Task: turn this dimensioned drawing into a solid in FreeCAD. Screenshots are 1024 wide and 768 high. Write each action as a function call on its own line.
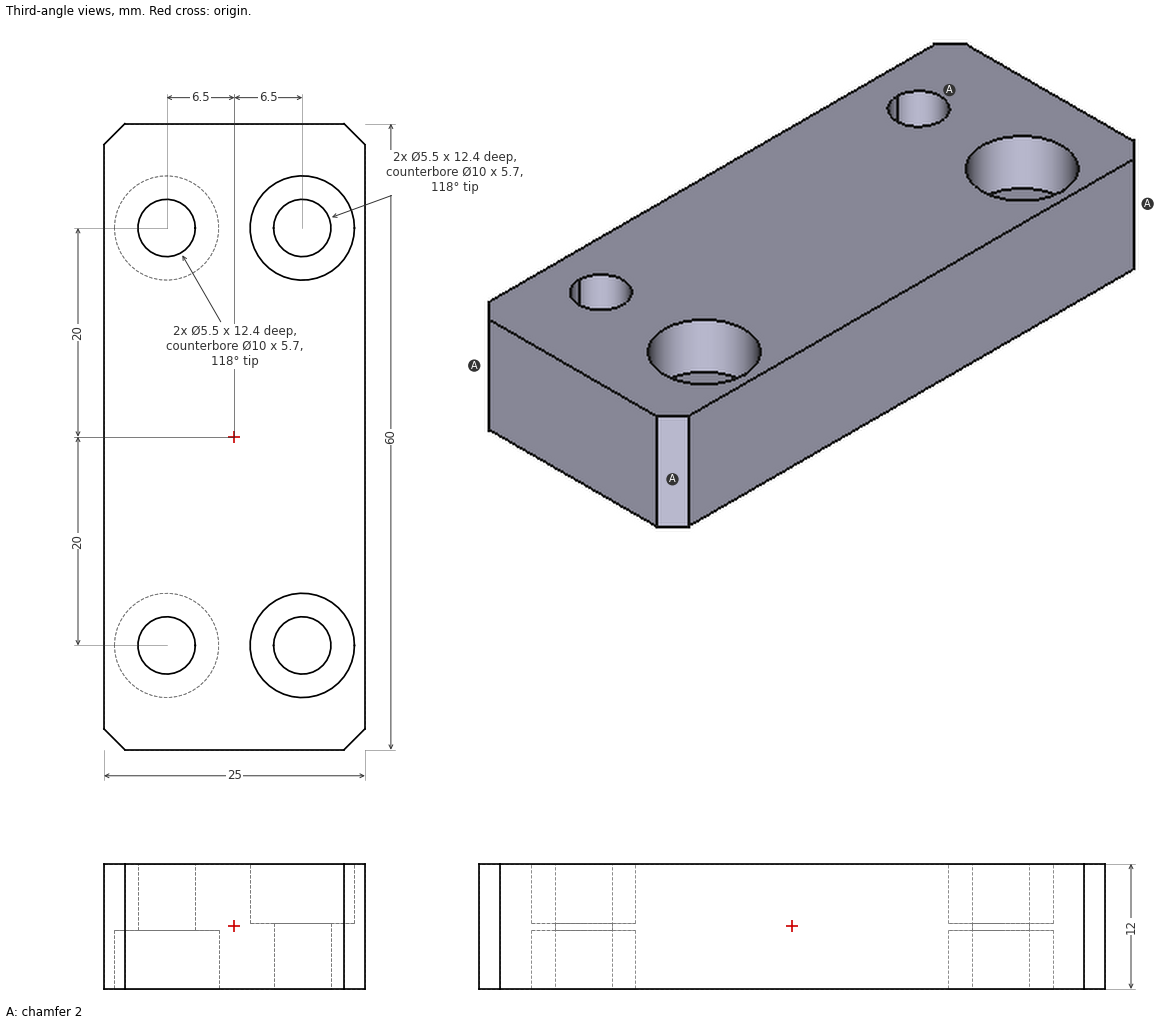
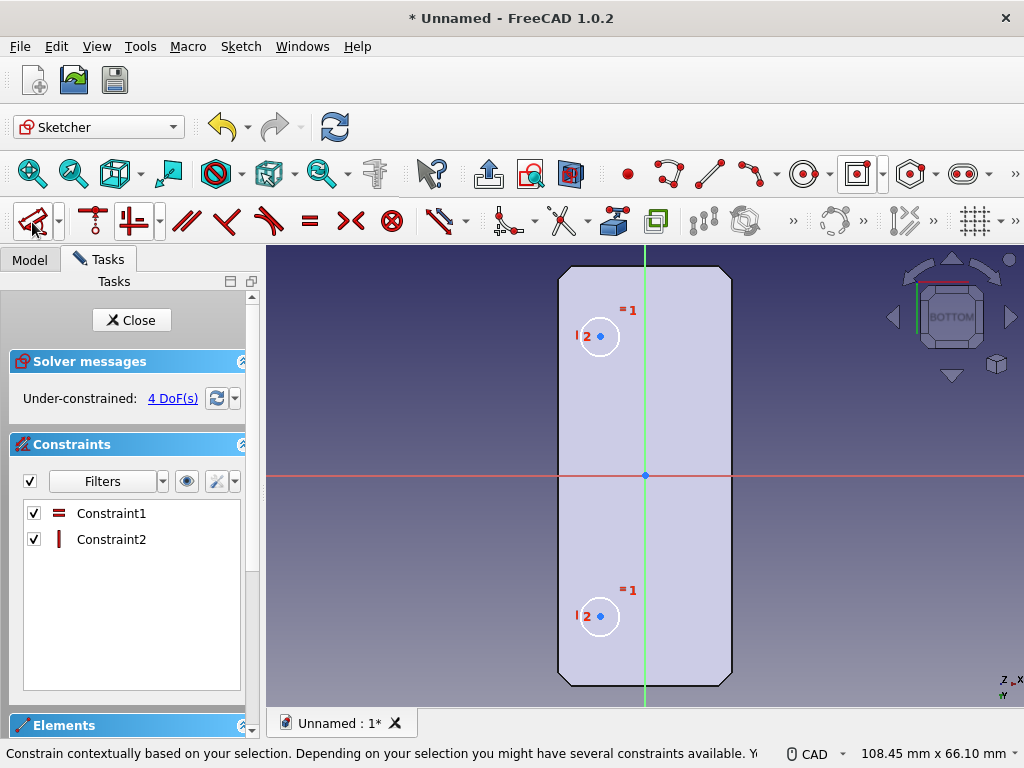
click(613, 603)
click(613, 567)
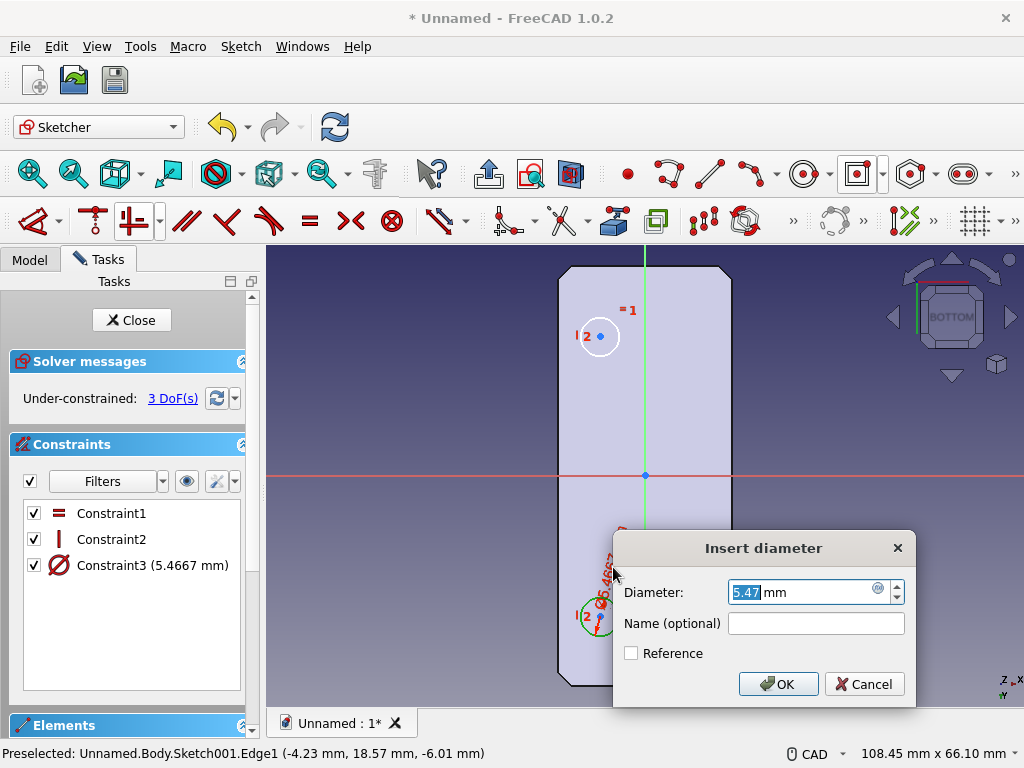
text(5.5)
key(Return)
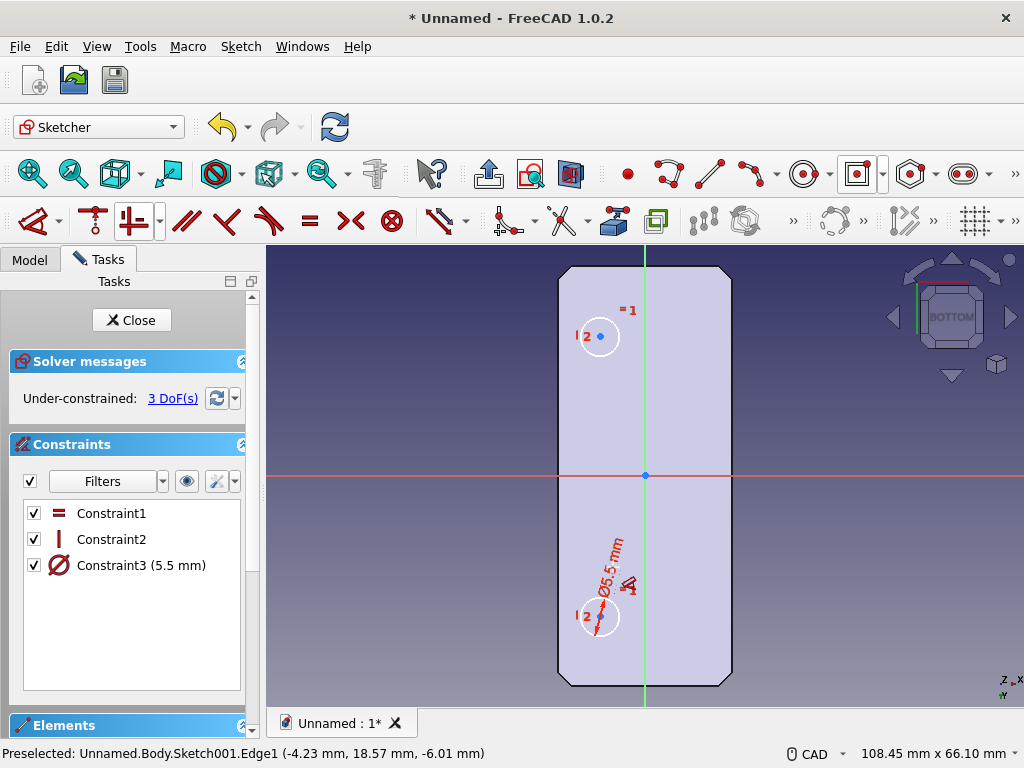
click(600, 617)
click(679, 547)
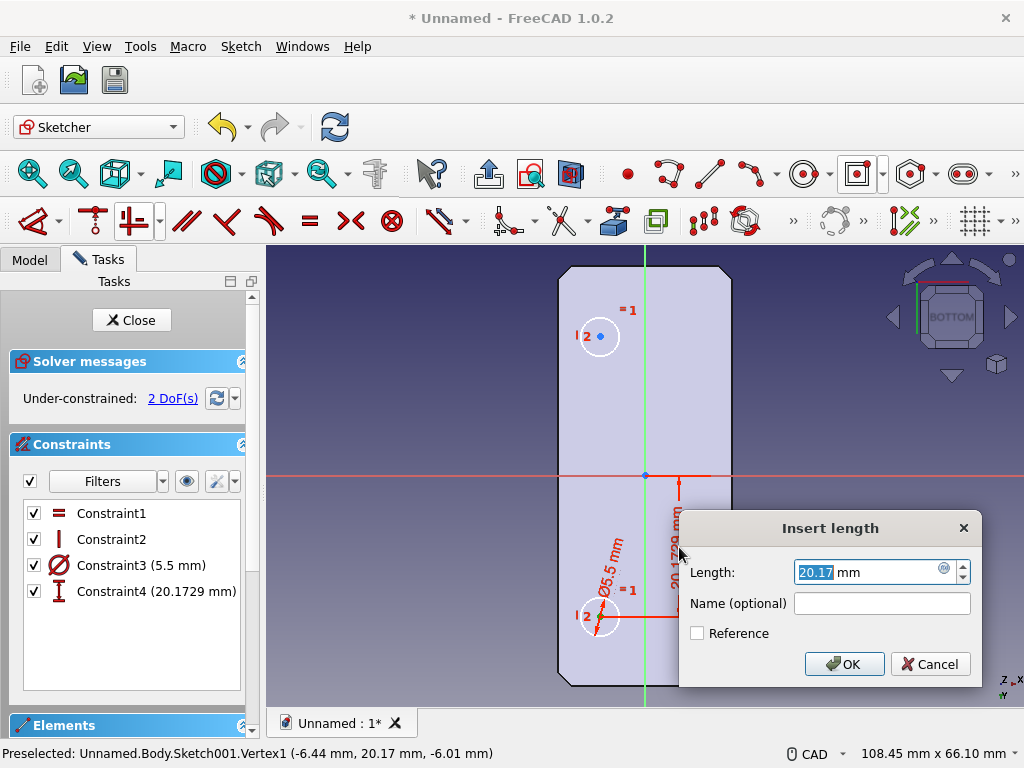
text(20)
key(Return)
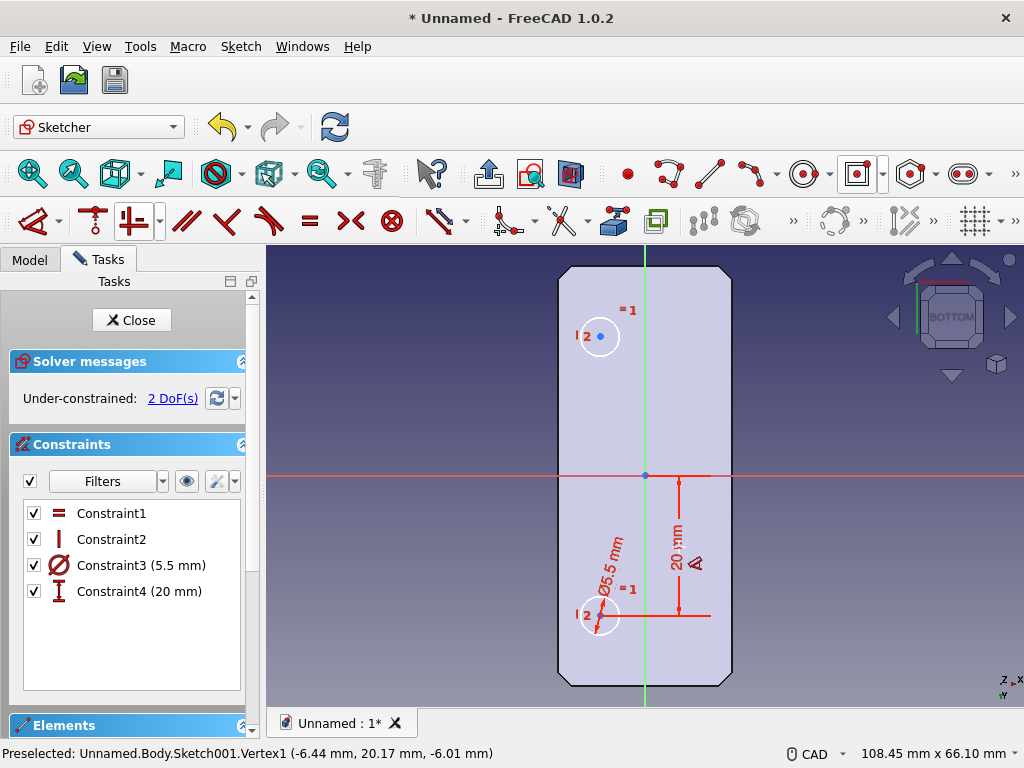
click(600, 337)
click(679, 406)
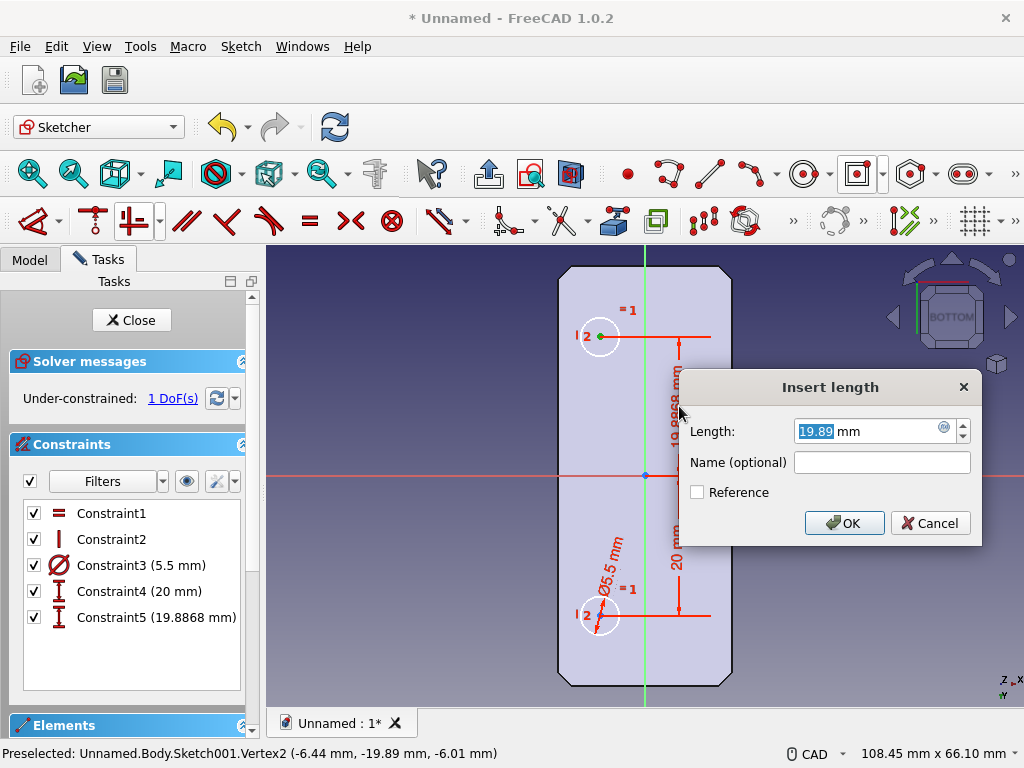
text(20)
key(Return)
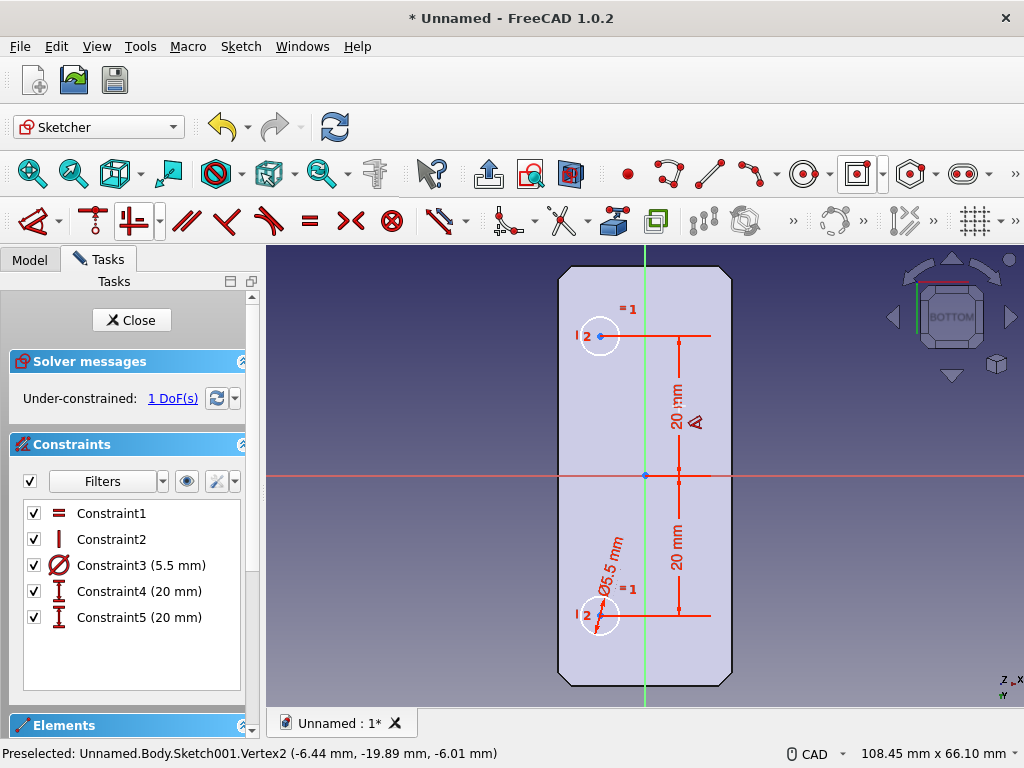
click(600, 616)
click(622, 650)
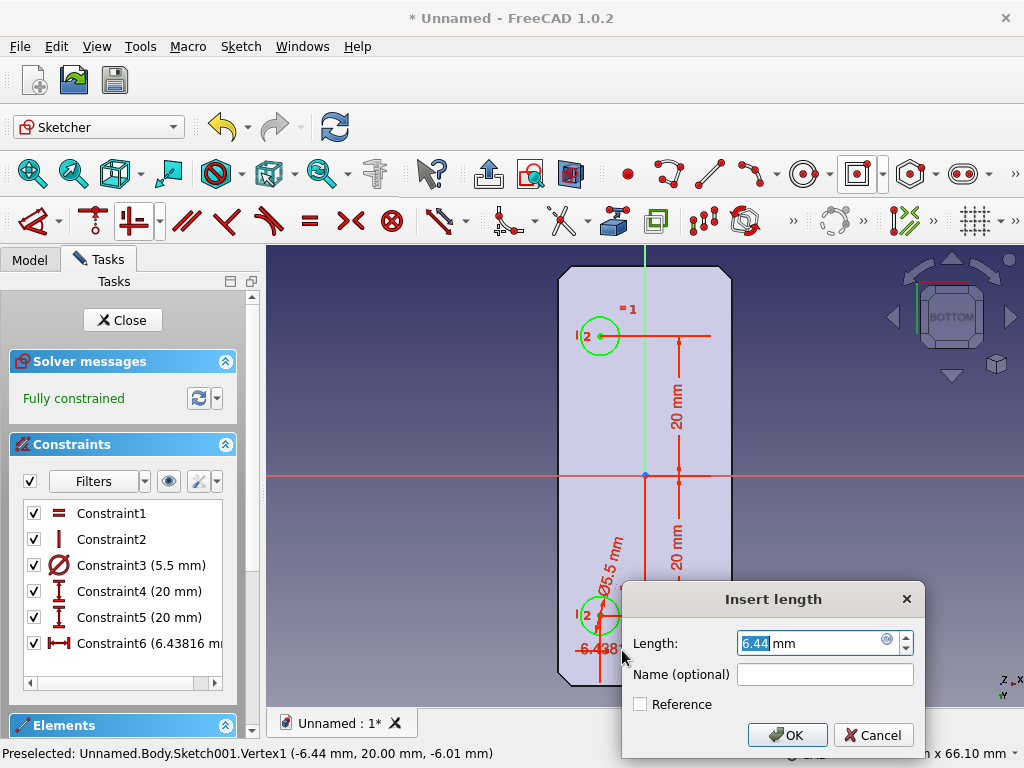
text(6.5)
key(Return)
key(Escape)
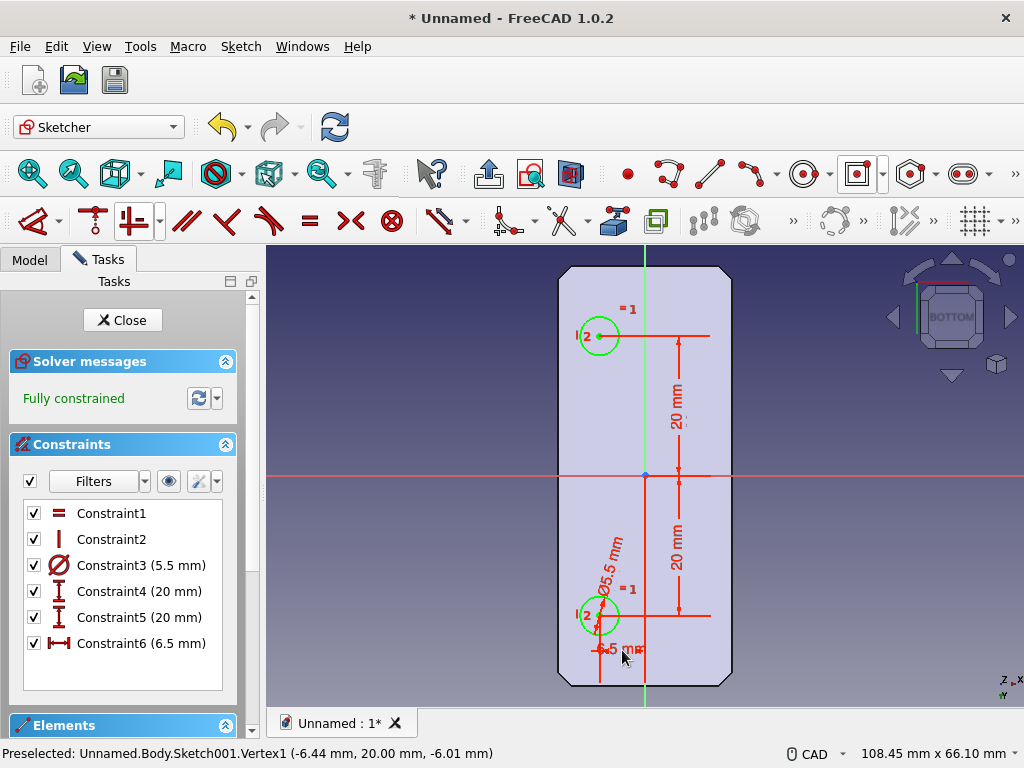
click(123, 320)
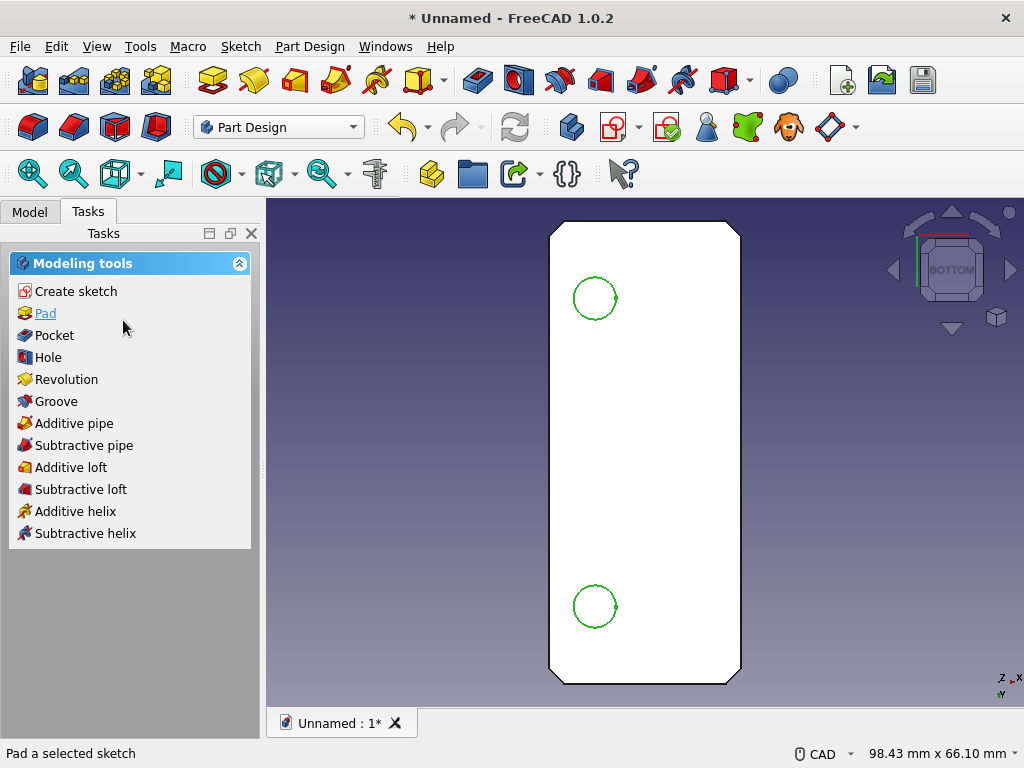
click(519, 80)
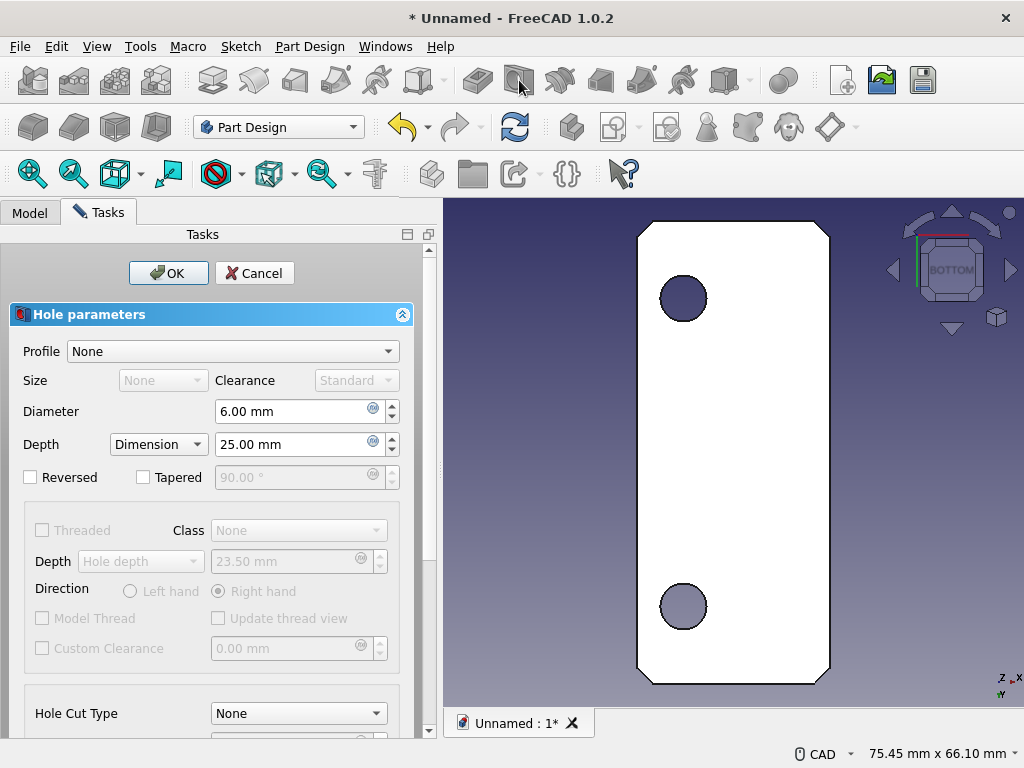
triple_click(300, 412)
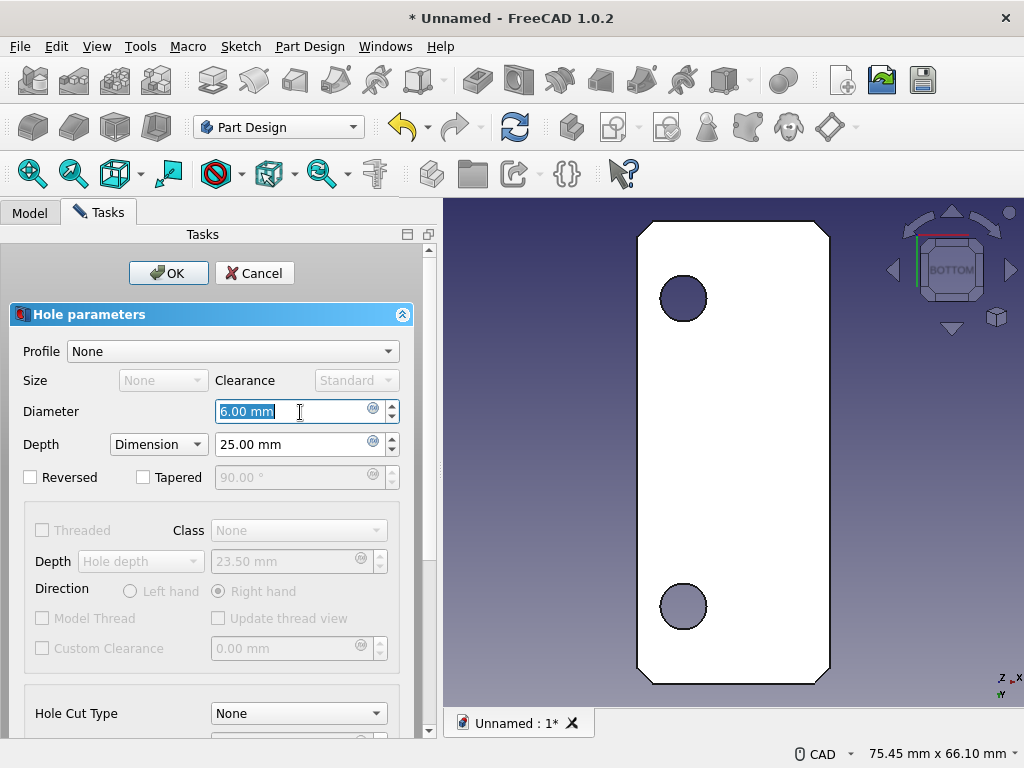
text(5.5)
key(Tab)